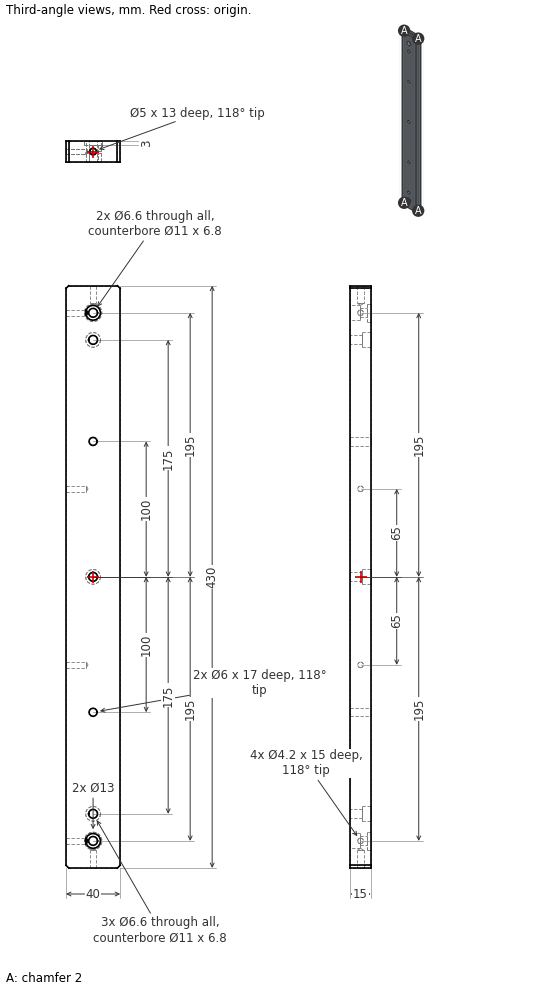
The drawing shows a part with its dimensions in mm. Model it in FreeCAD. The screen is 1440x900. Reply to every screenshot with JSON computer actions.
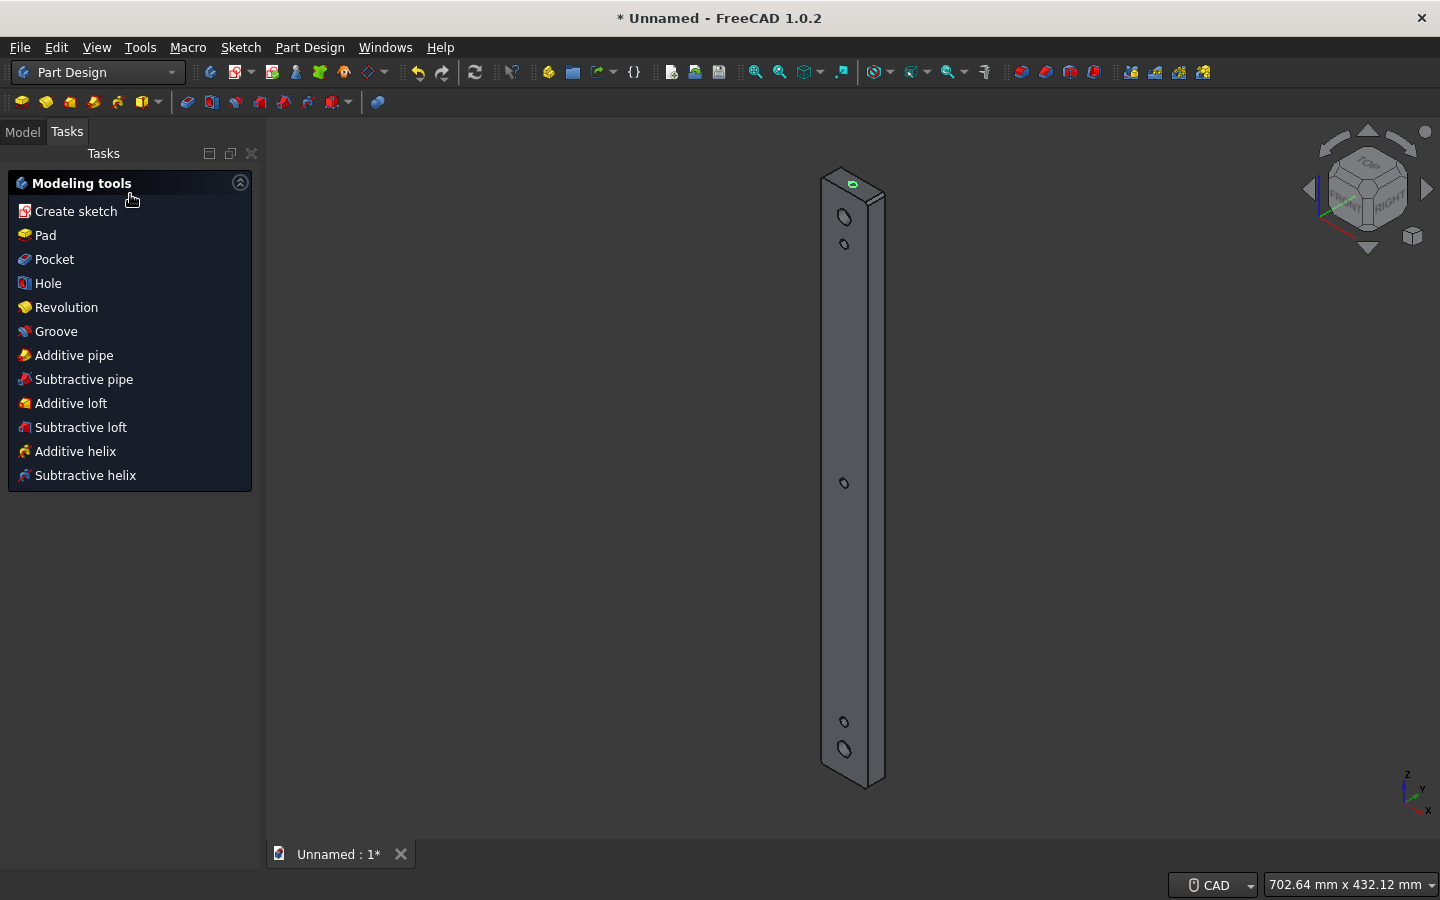
{"action": "left_click", "coordinate": [212, 102]}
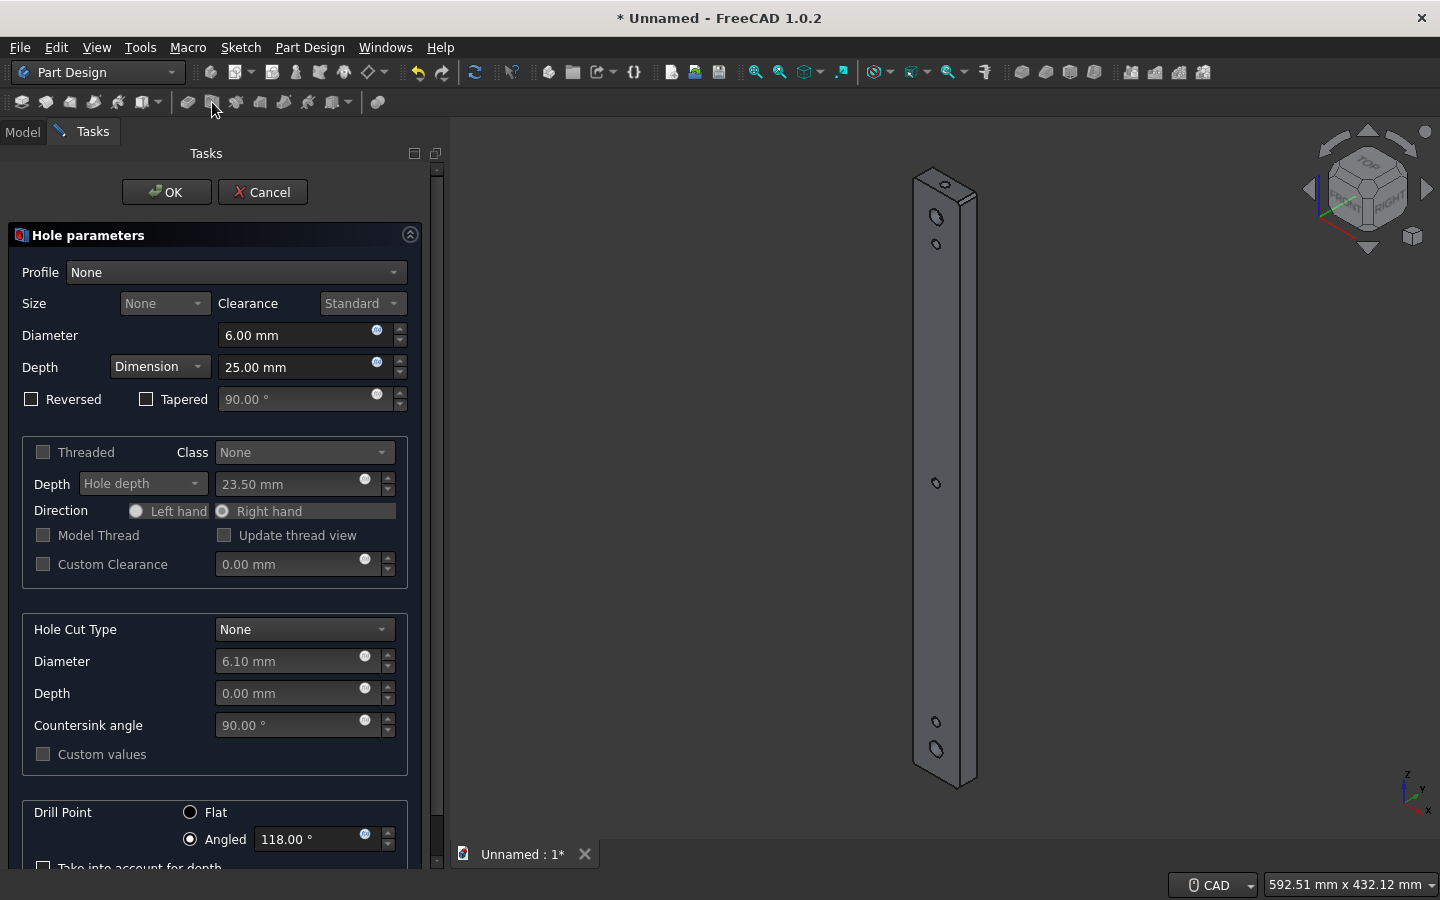
{"action": "triple_click", "coordinate": [305, 335]}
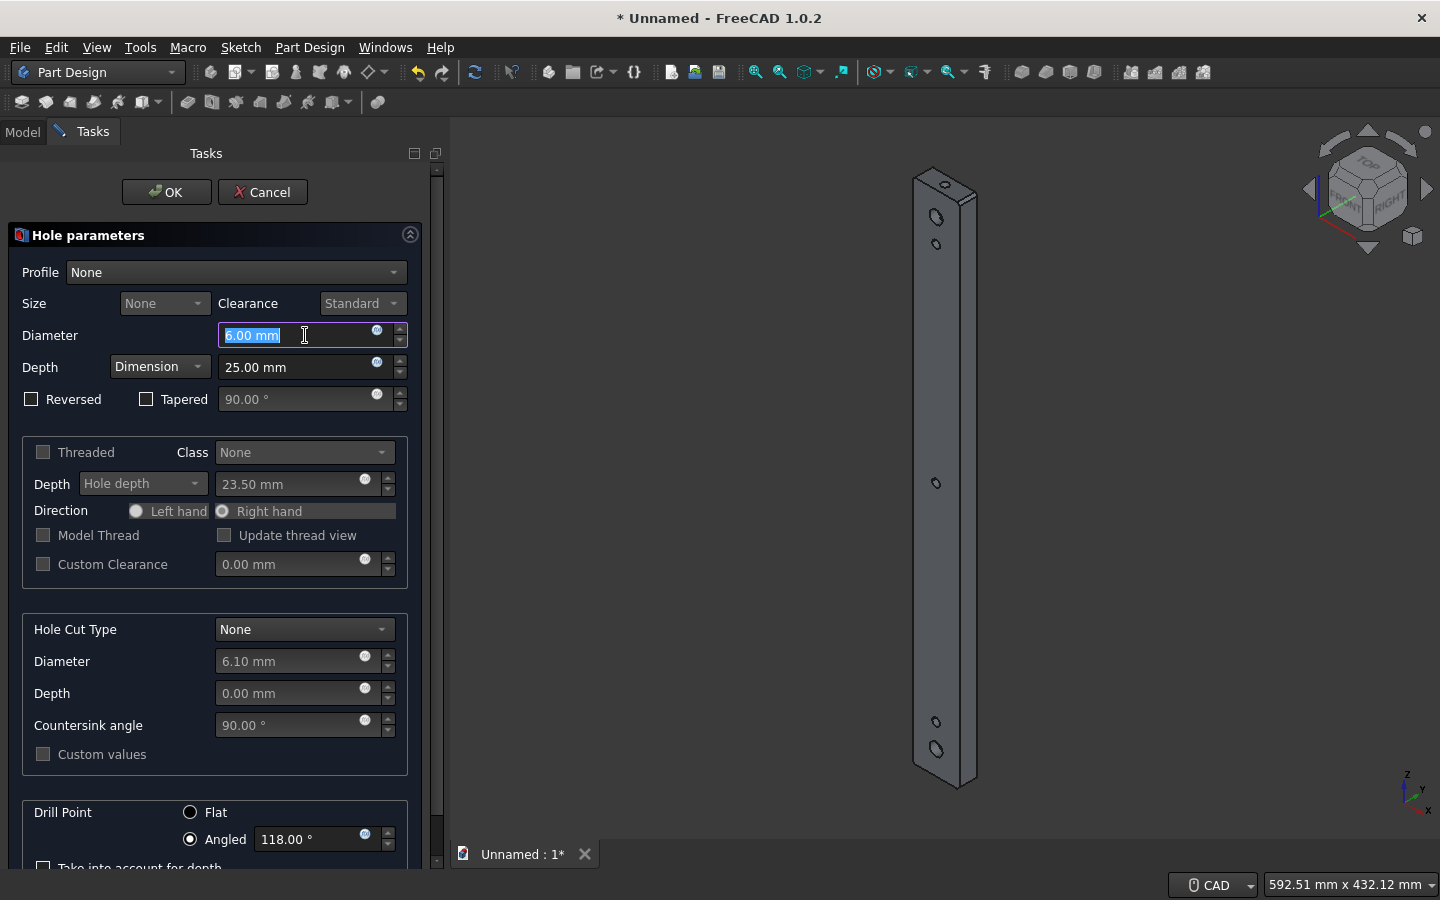
{"action": "type", "text": "5"}
{"action": "key", "text": "Tab"}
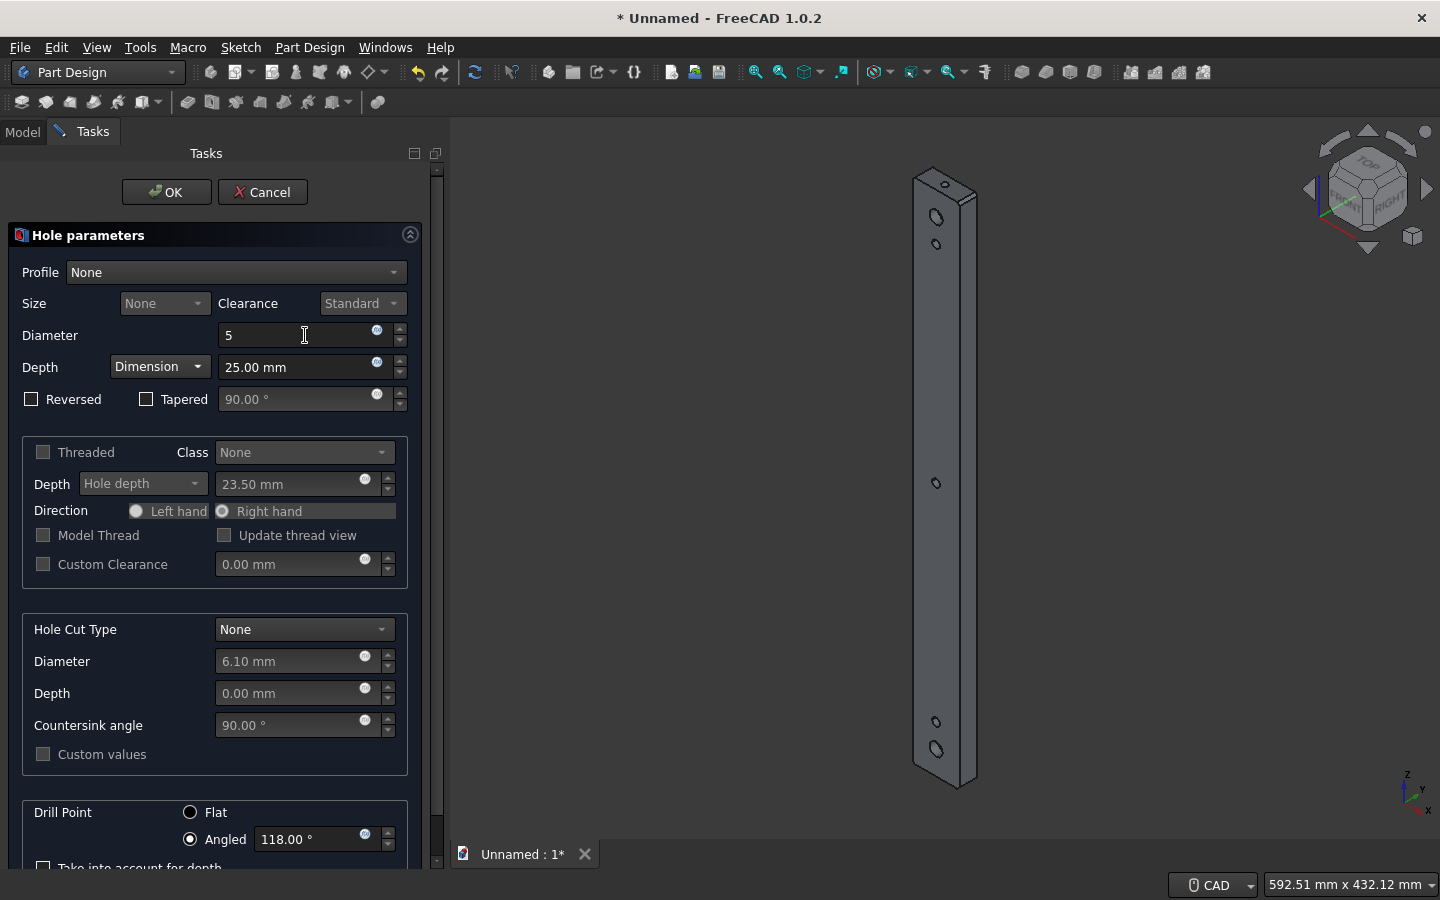
{"action": "triple_click", "coordinate": [305, 367]}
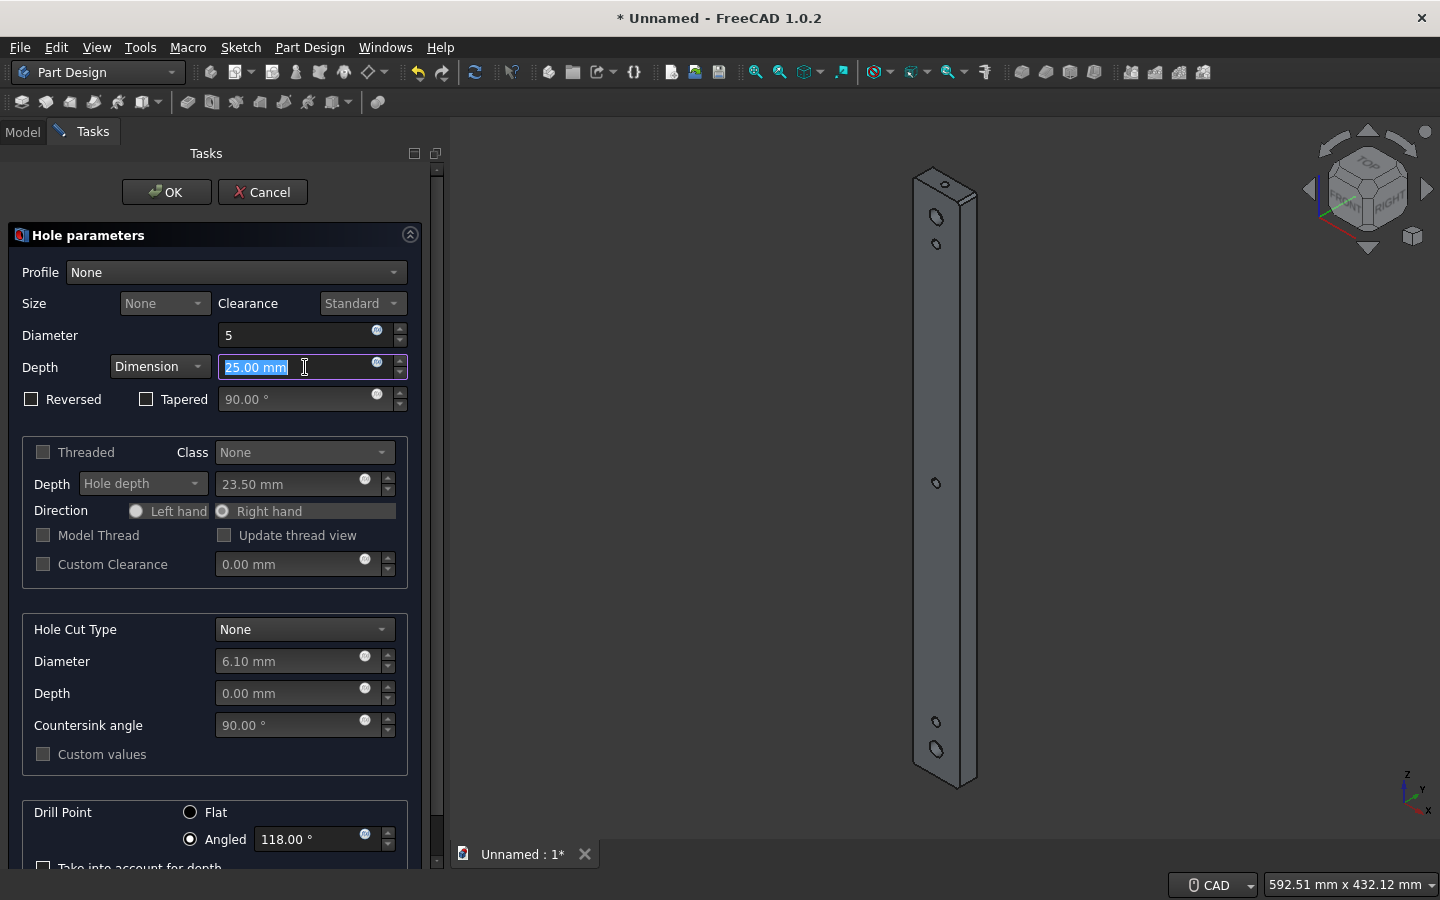
{"action": "type", "text": "13"}
{"action": "key", "text": "Tab"}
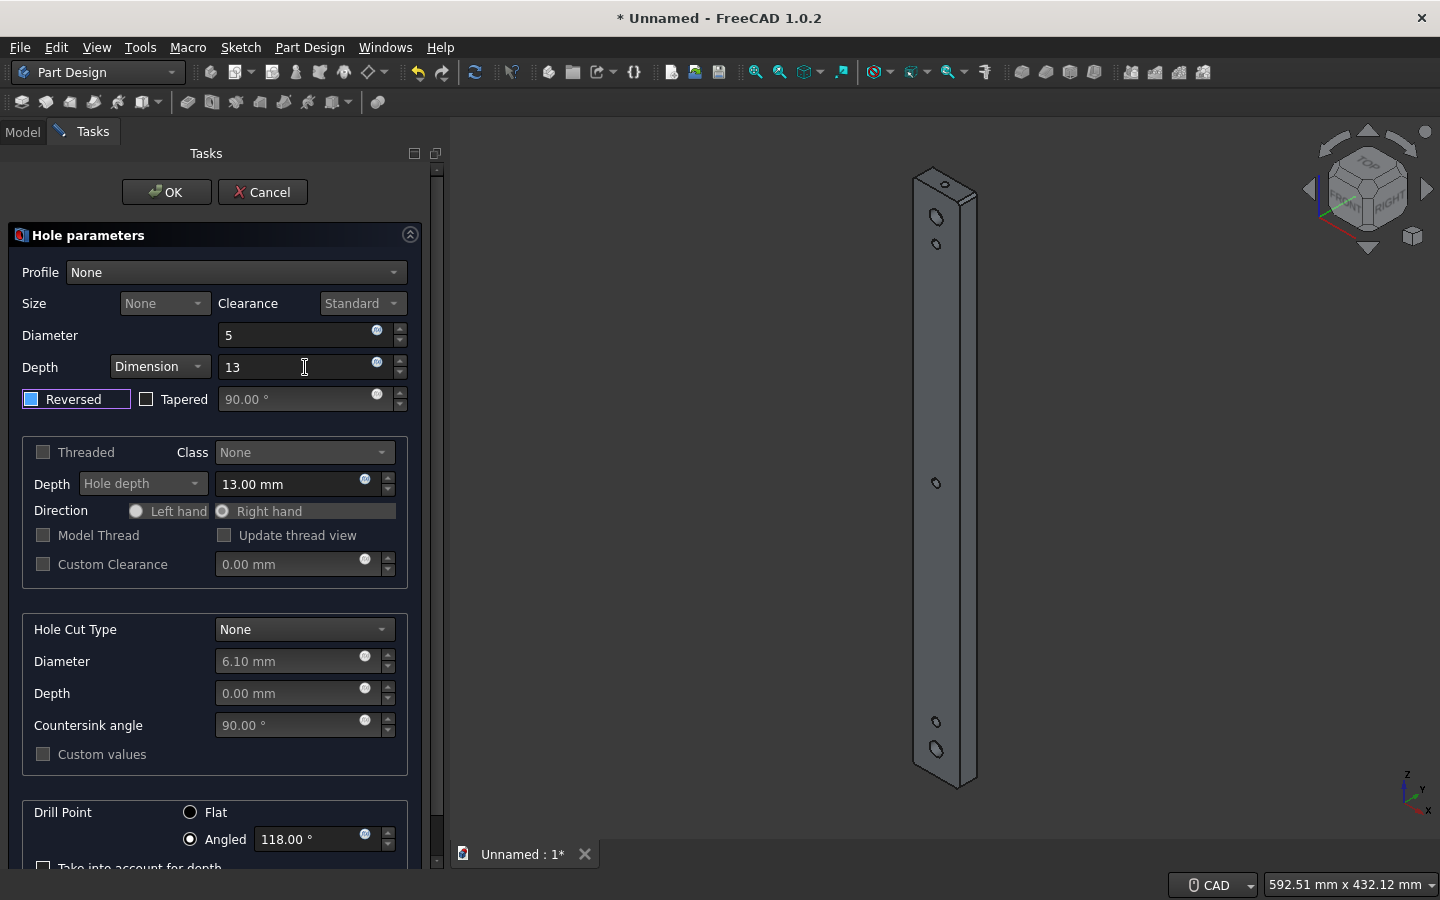
{"action": "left_click", "coordinate": [167, 192]}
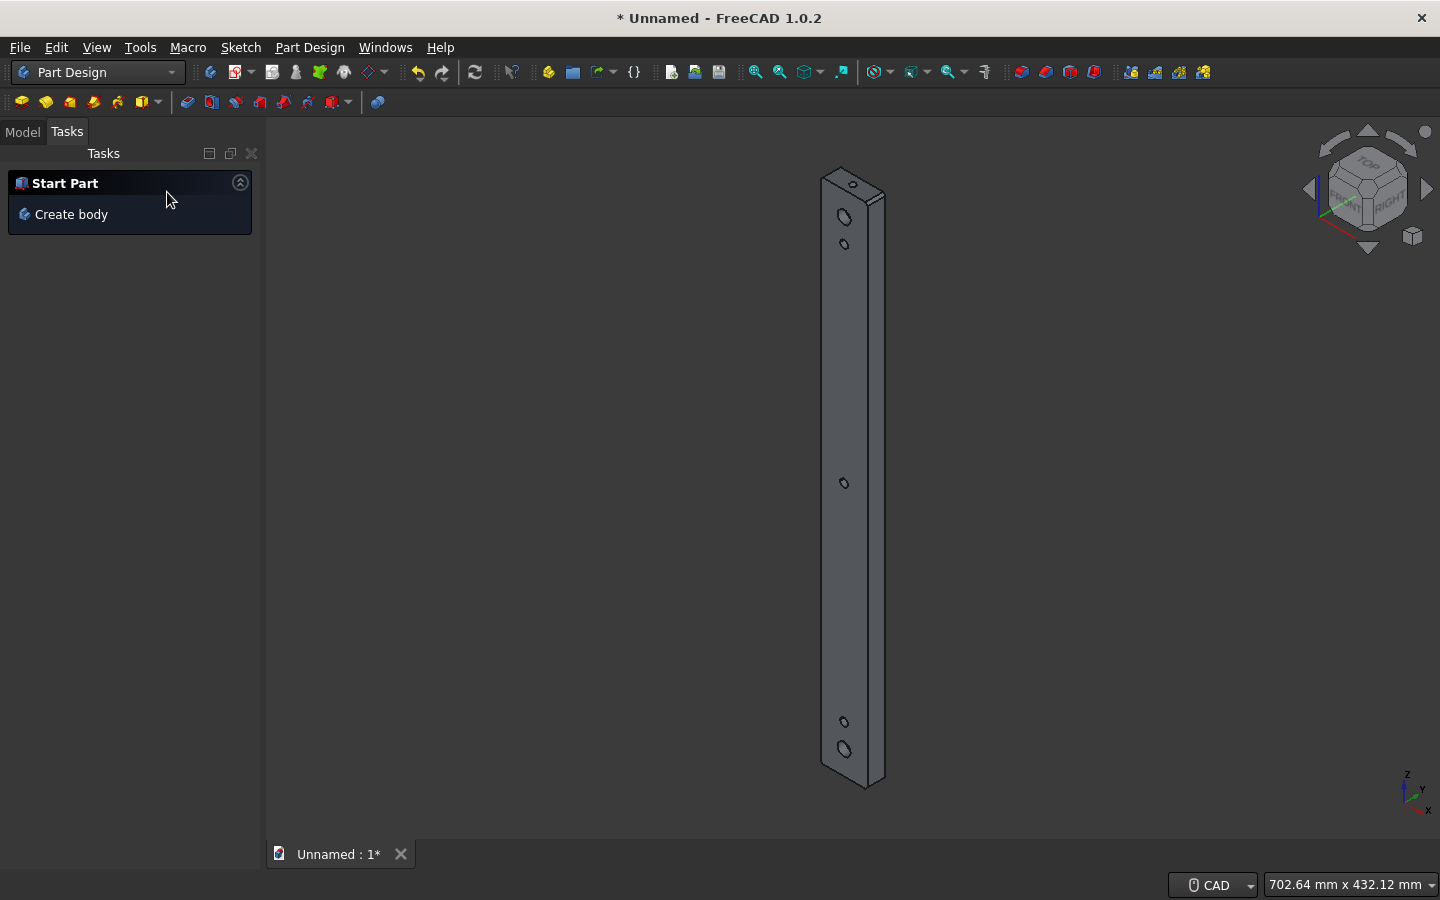
{"action": "key", "text": "5"}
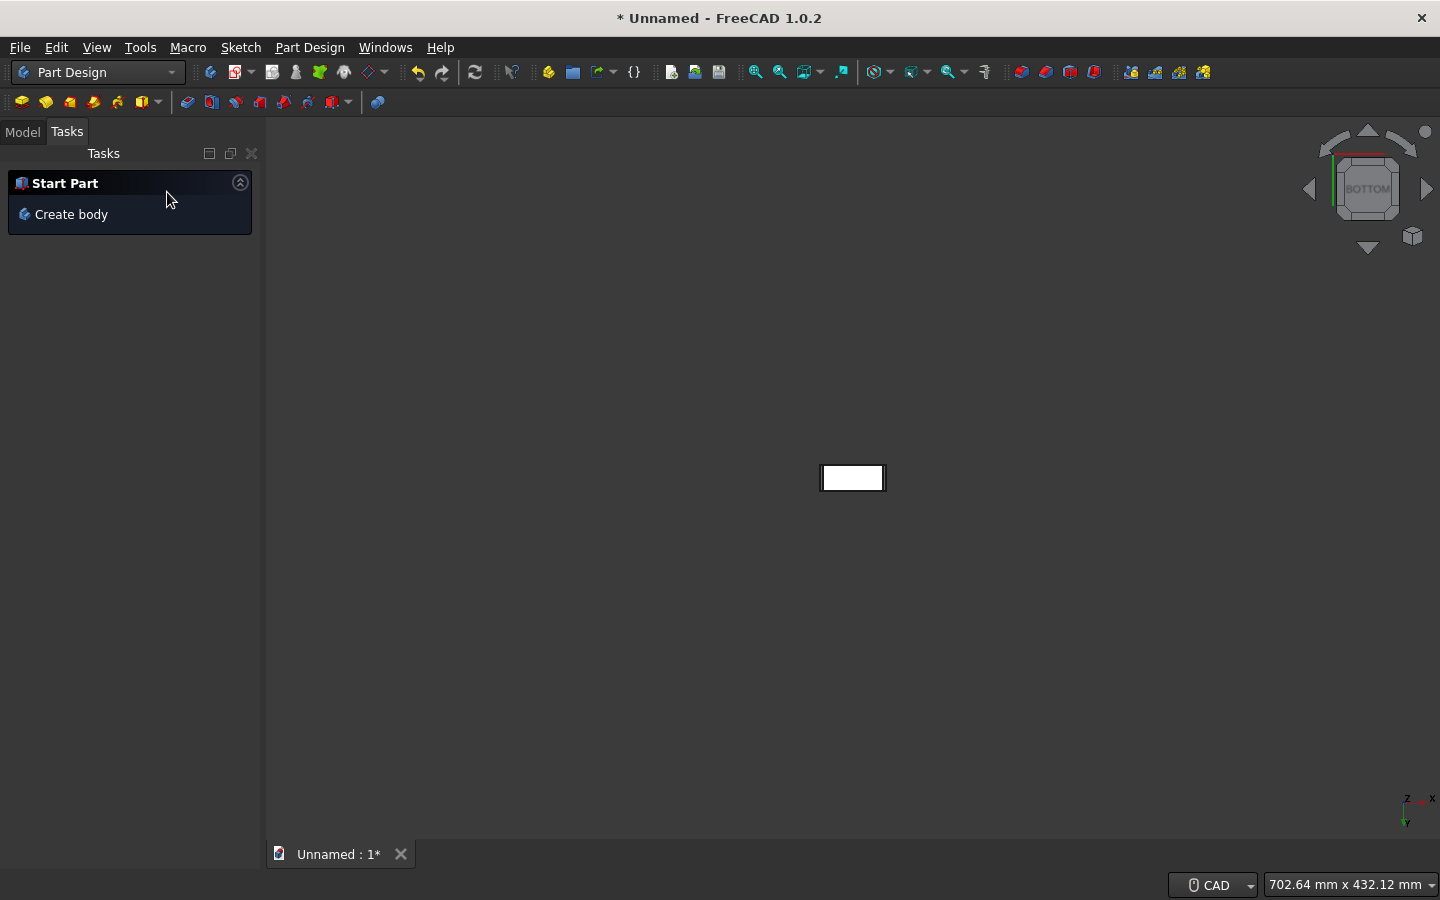
{"action": "key", "text": "v f"}